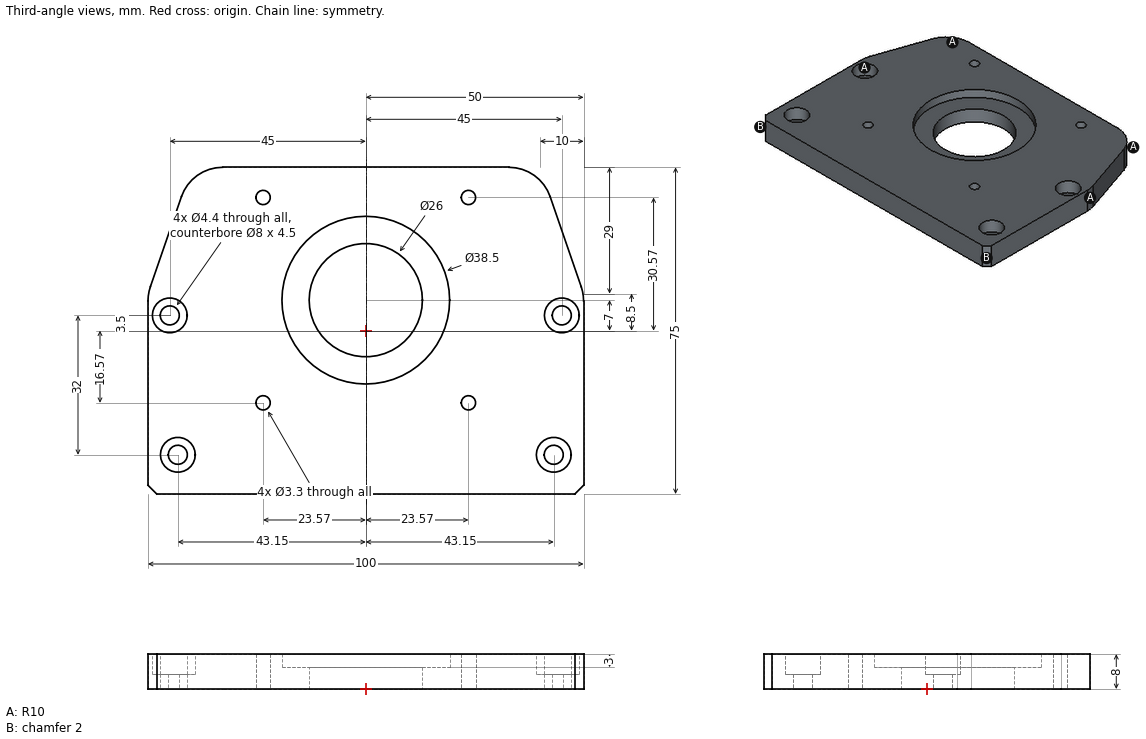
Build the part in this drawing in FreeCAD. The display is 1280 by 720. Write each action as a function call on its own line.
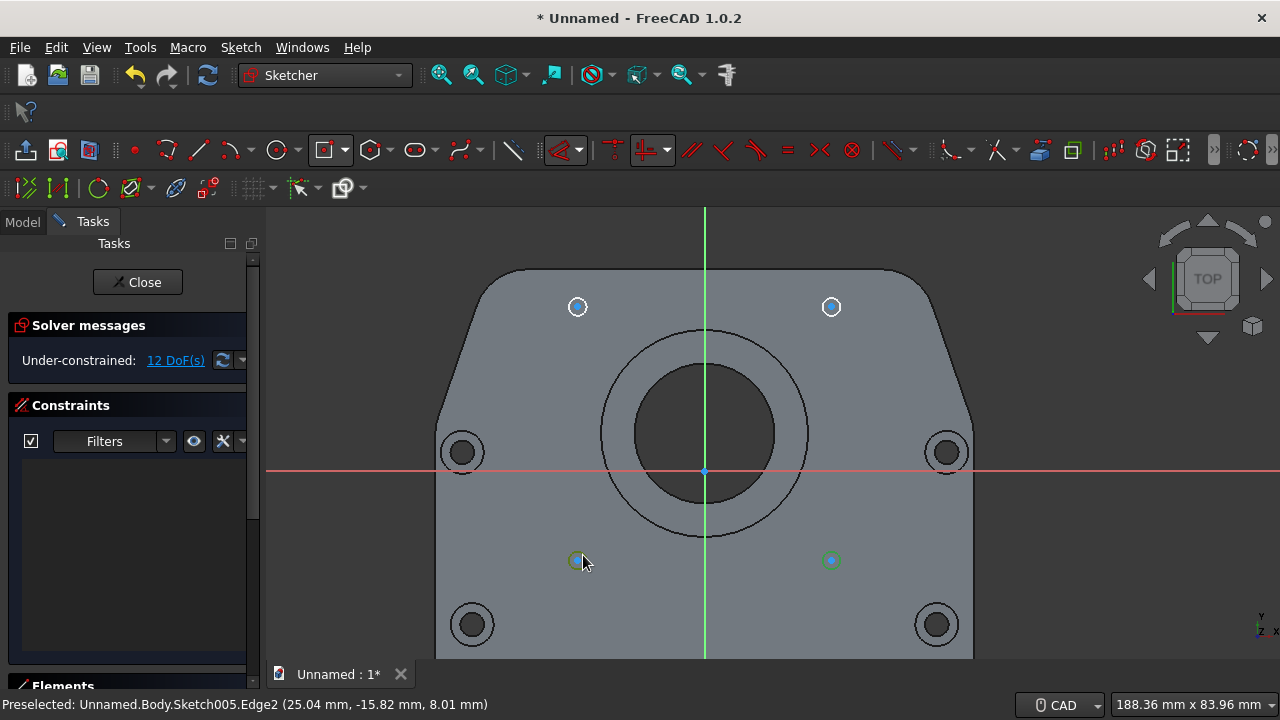
scroll(838, 301, up, 3)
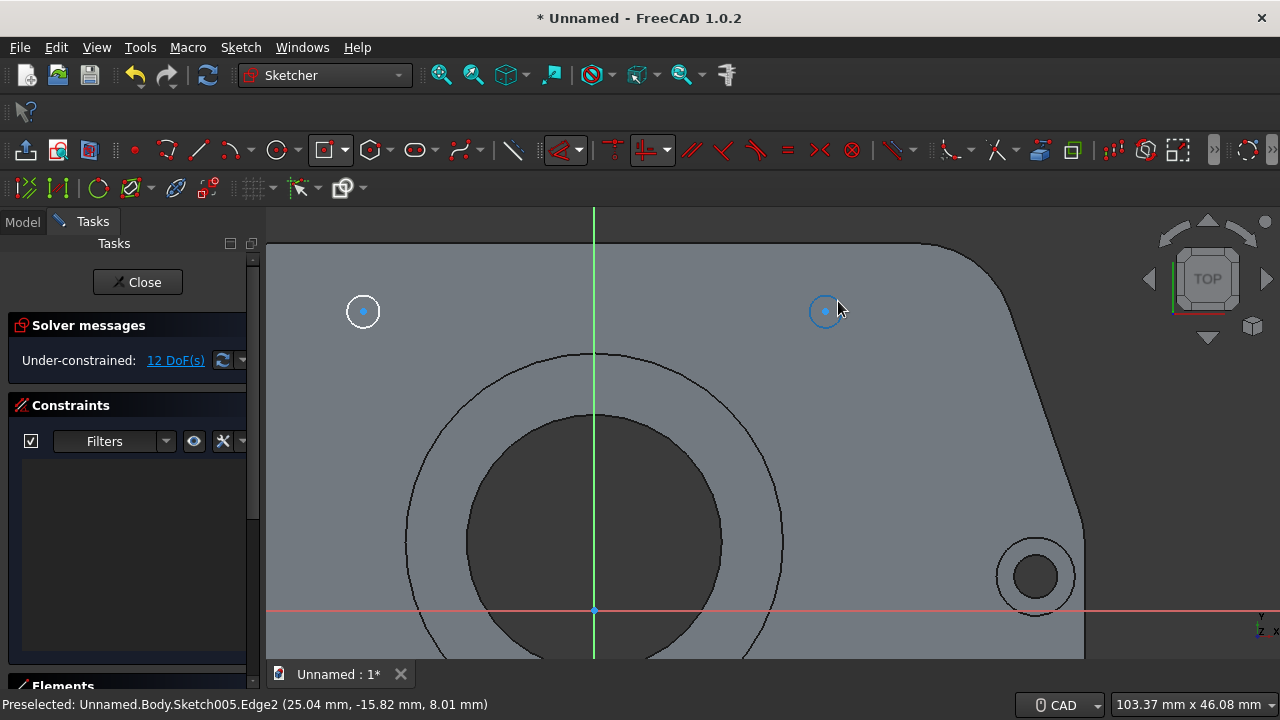
click(837, 300)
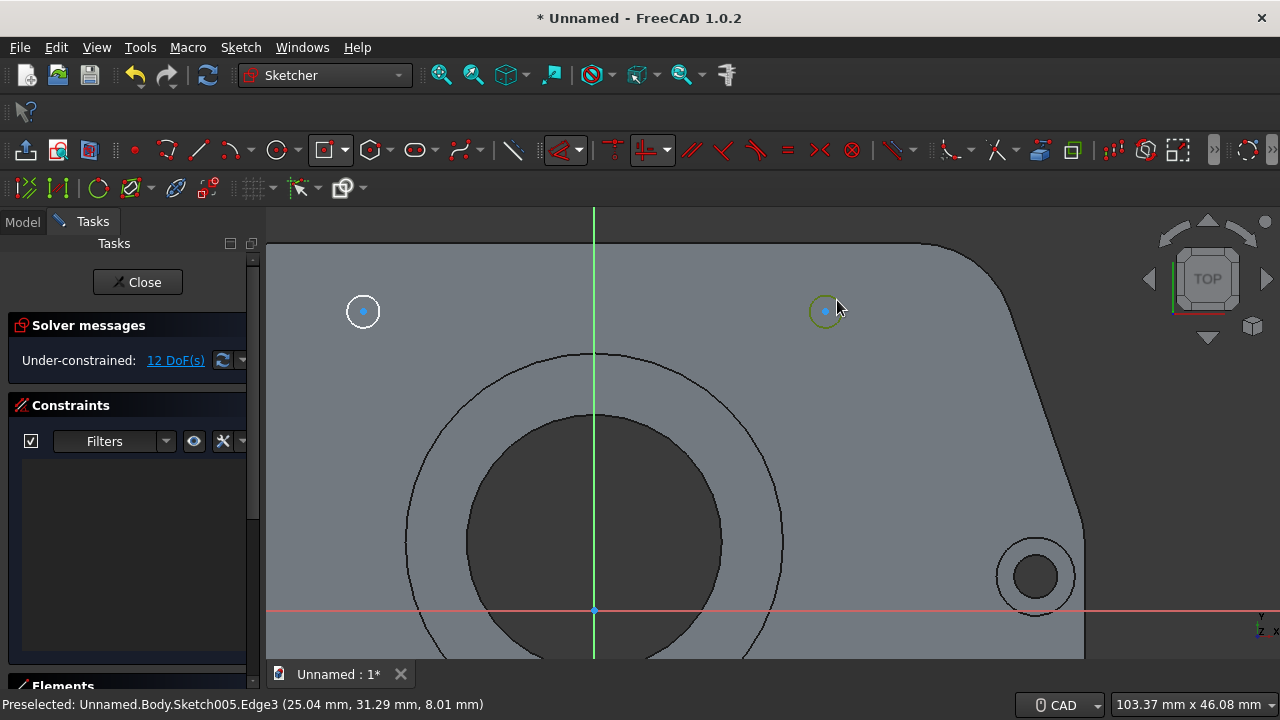
click(375, 300)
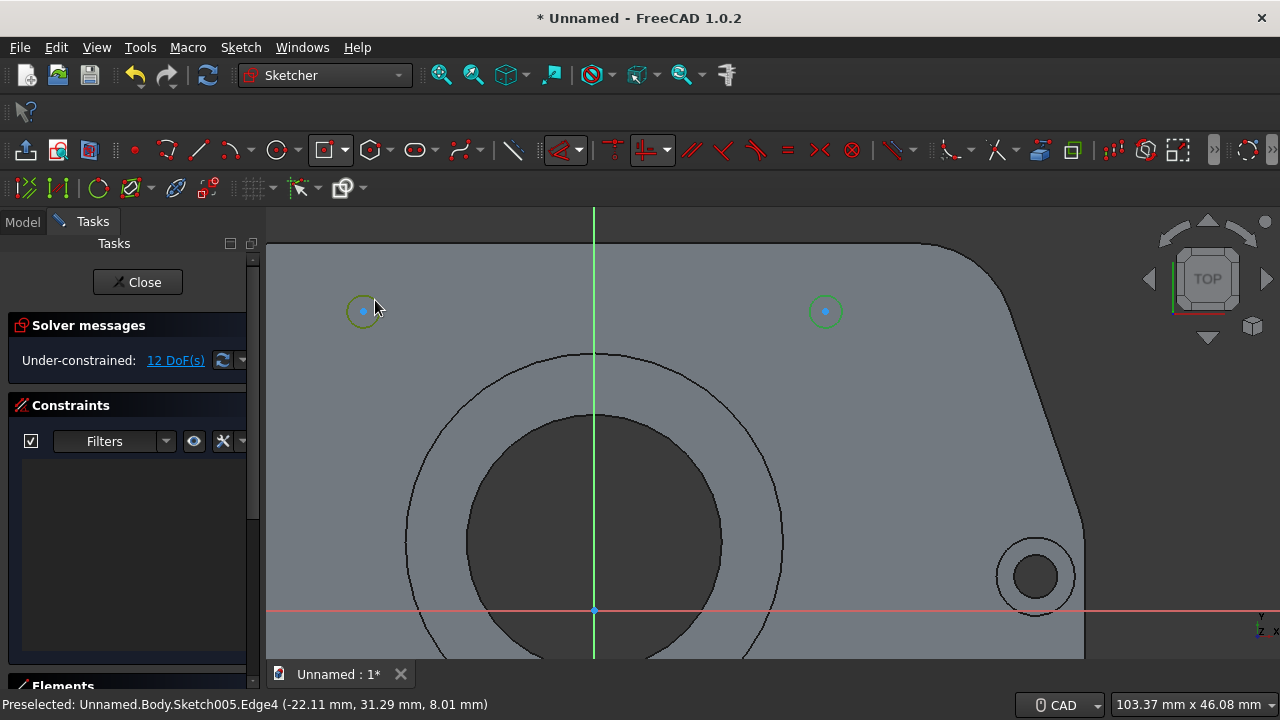
click(788, 150)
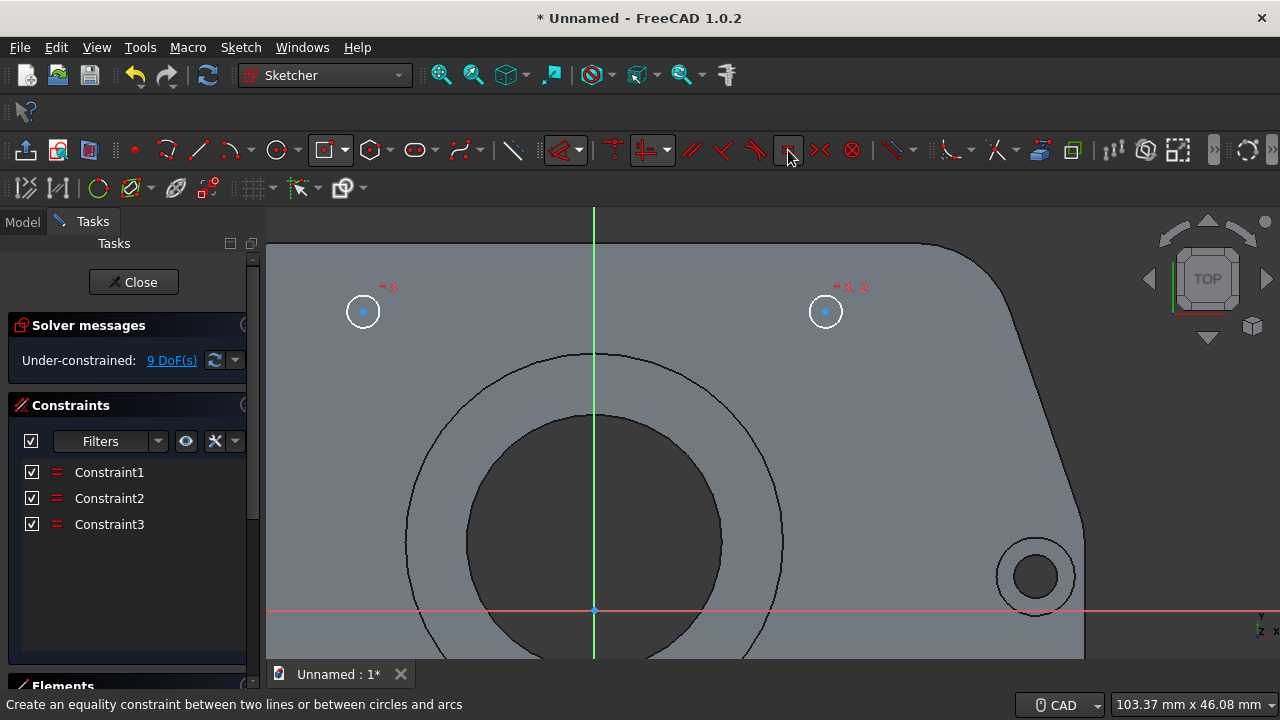
scroll(839, 300, down, 3)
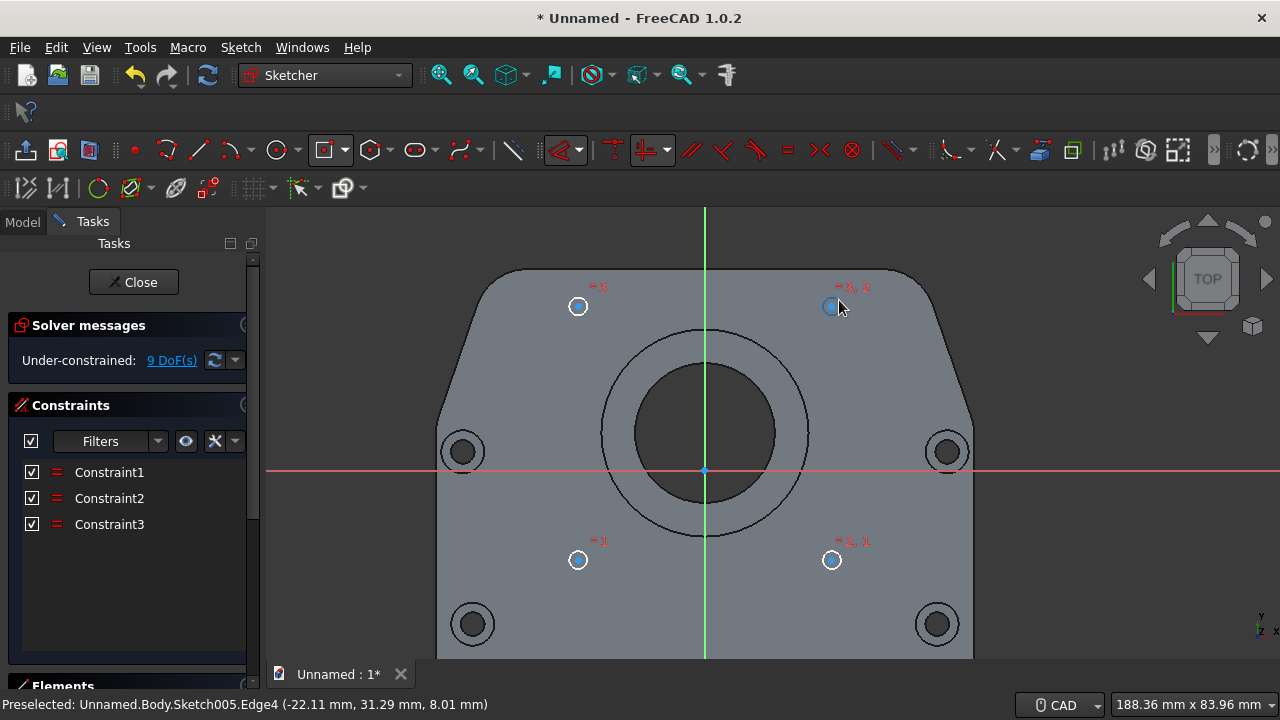
click(578, 560)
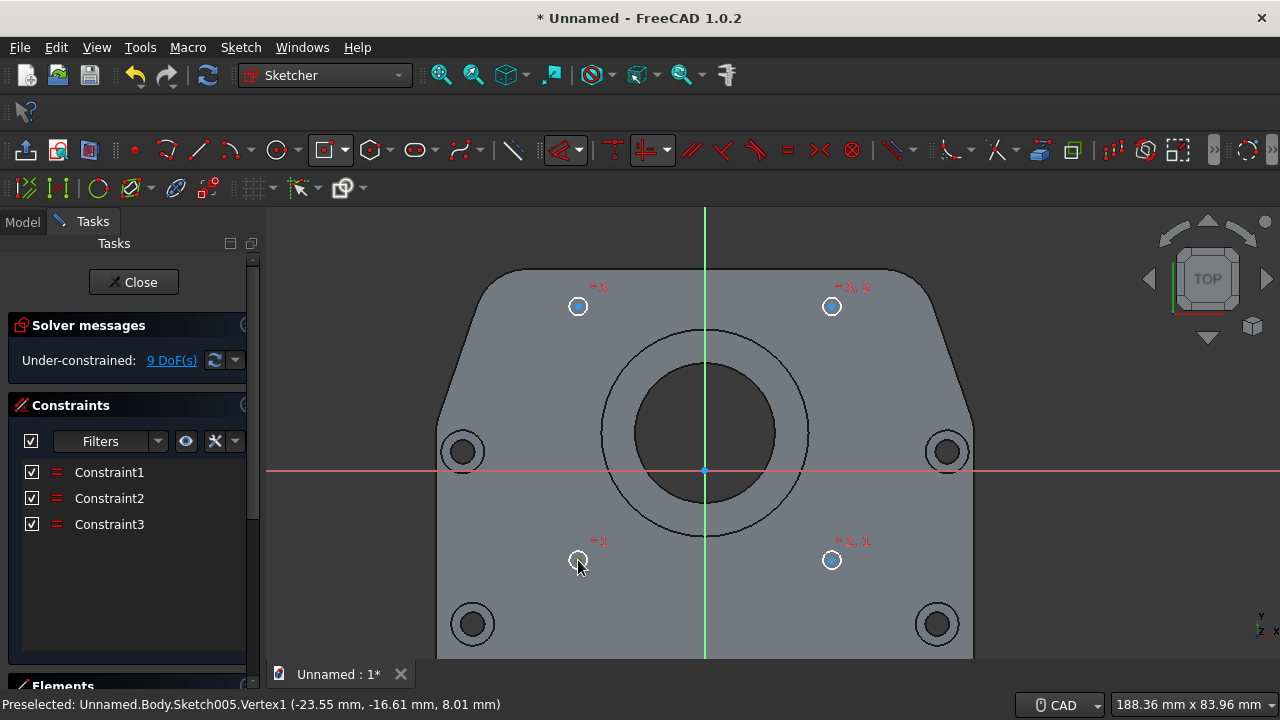
click(832, 560)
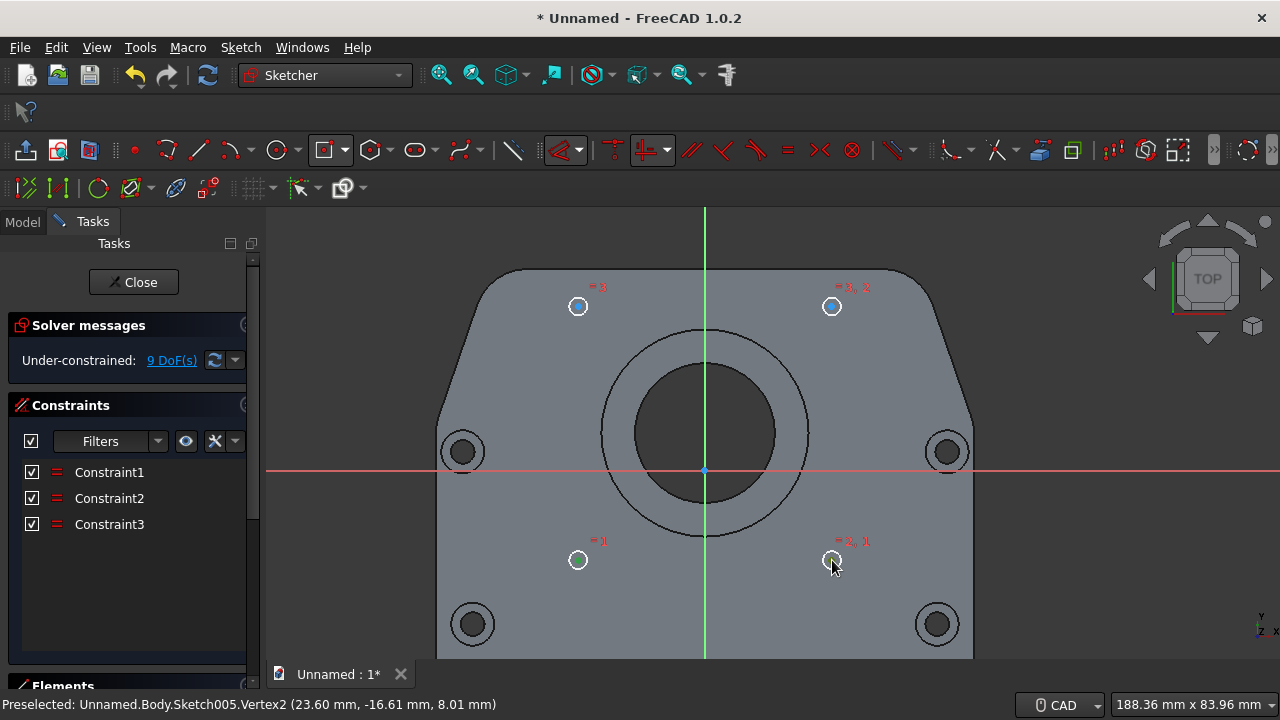
key(h)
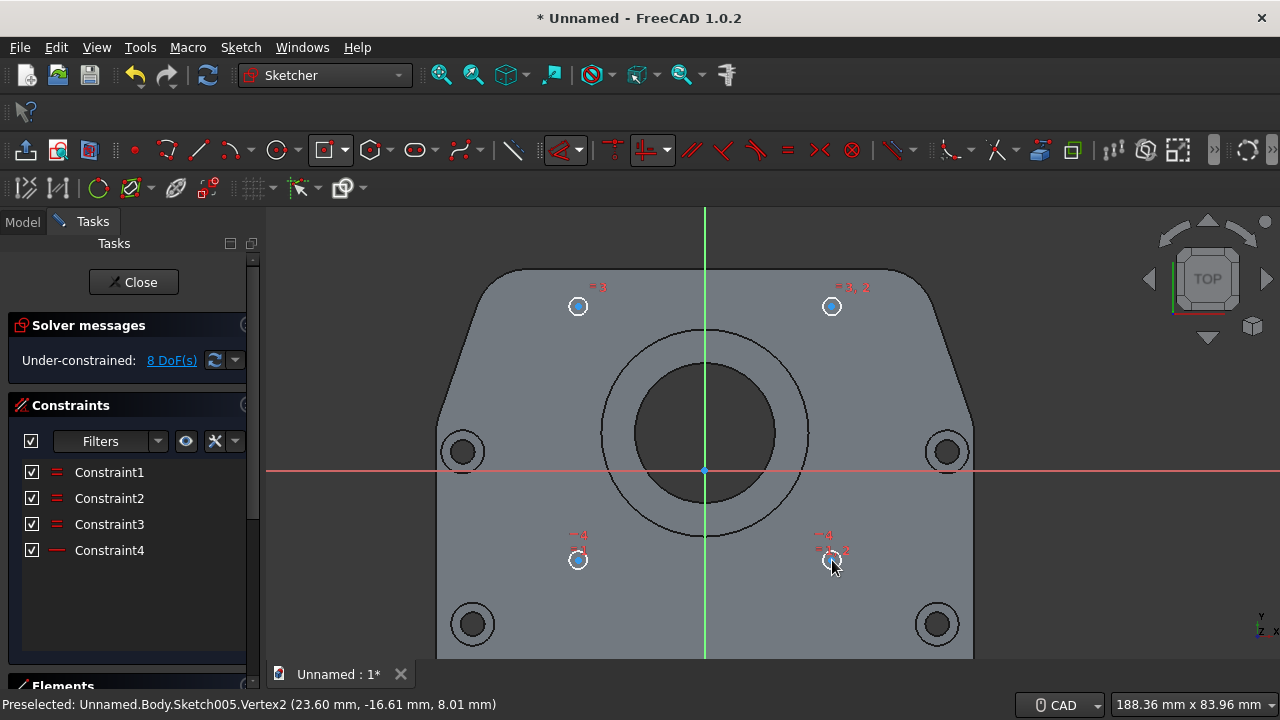
click(832, 560)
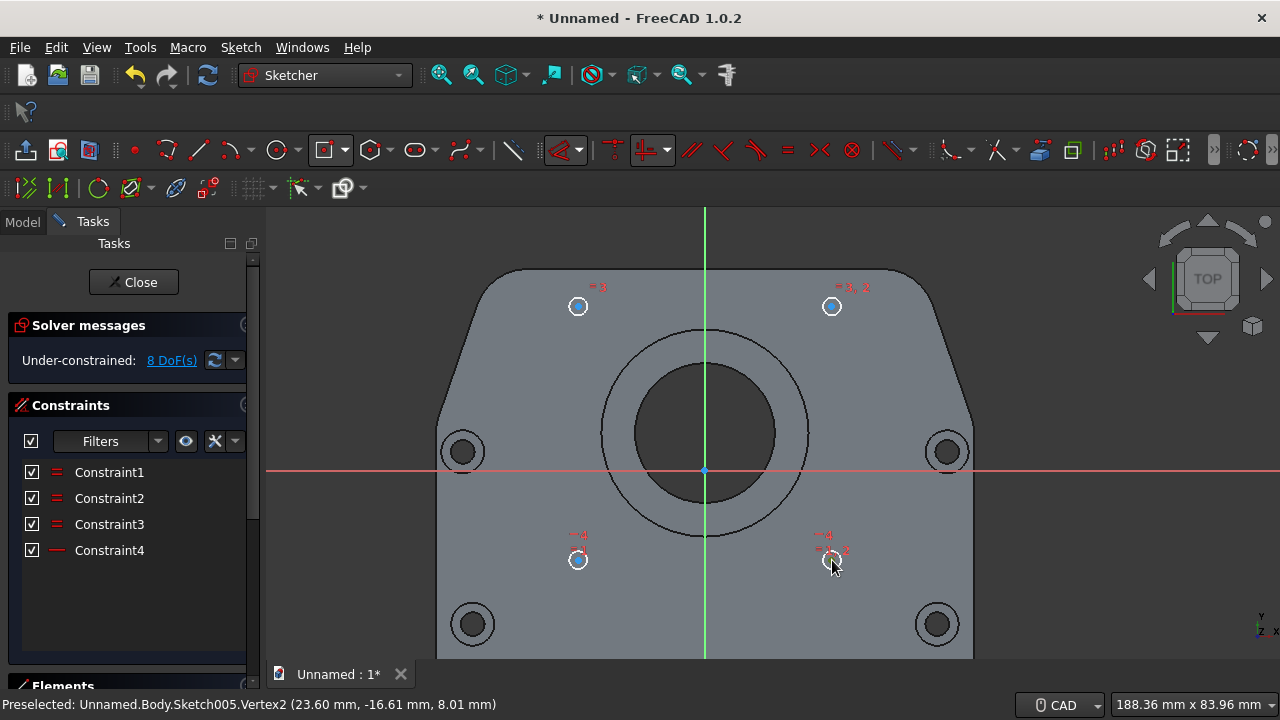
click(832, 307)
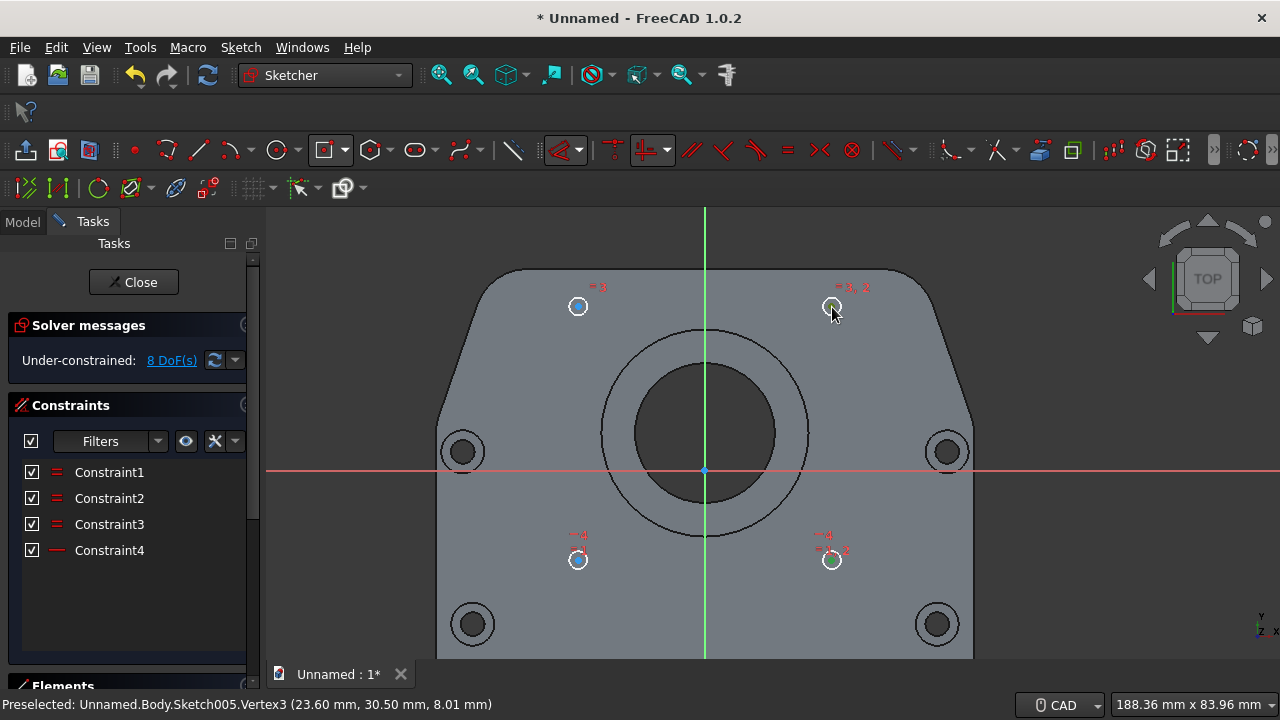
key(v)